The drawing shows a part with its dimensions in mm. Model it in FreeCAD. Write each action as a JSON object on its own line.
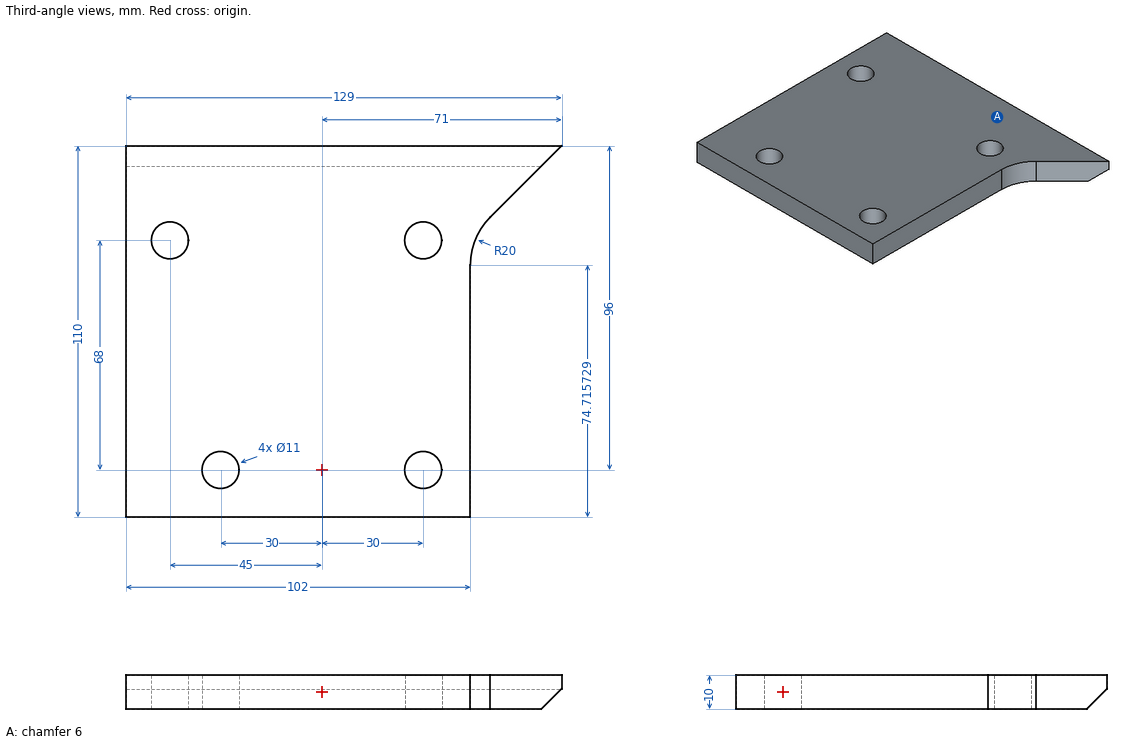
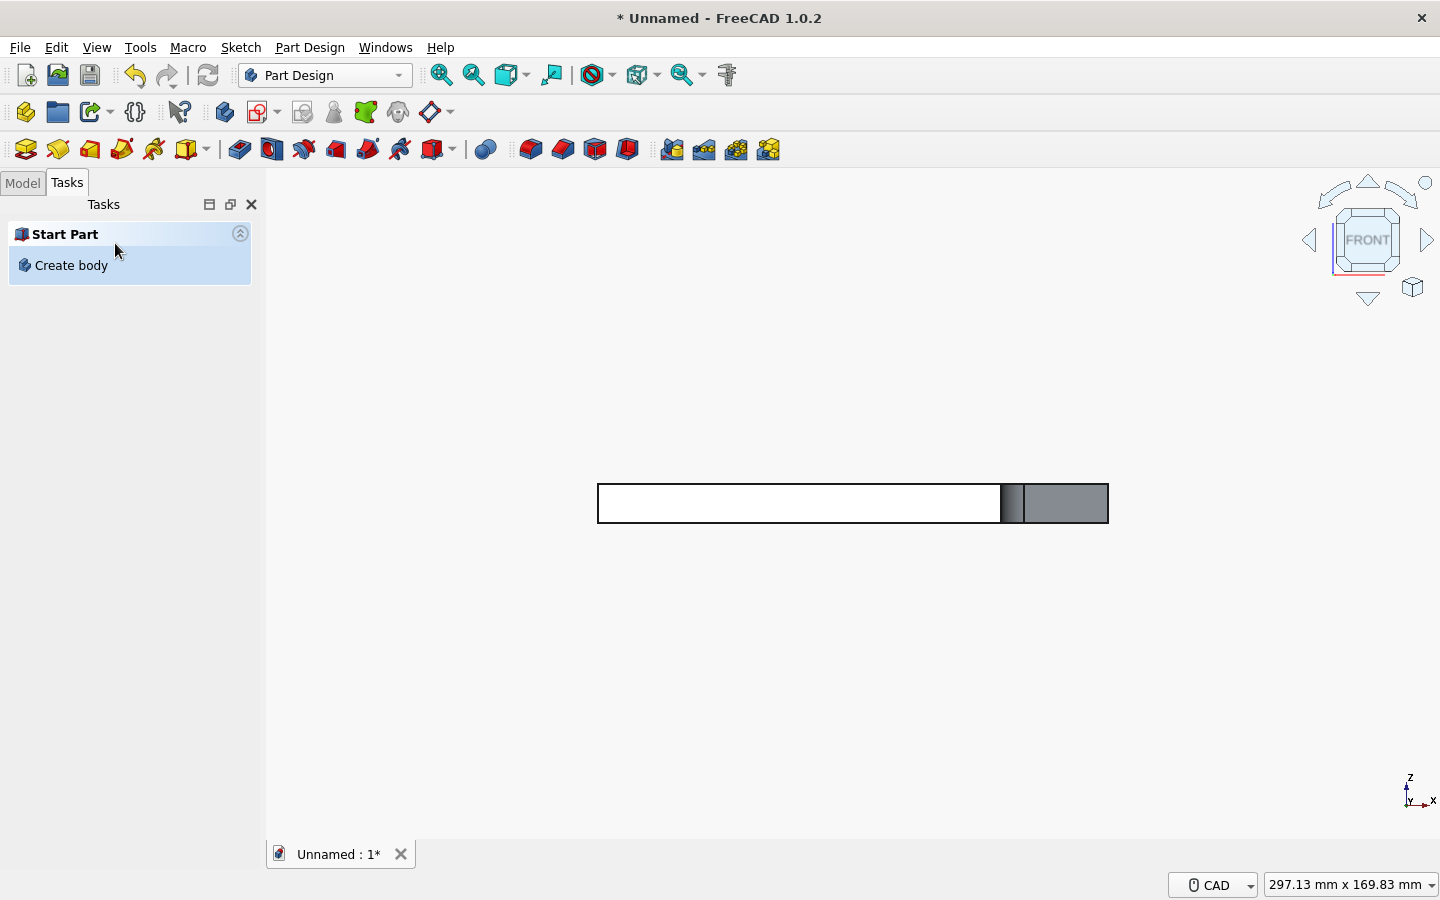
{"action": "key", "text": "3"}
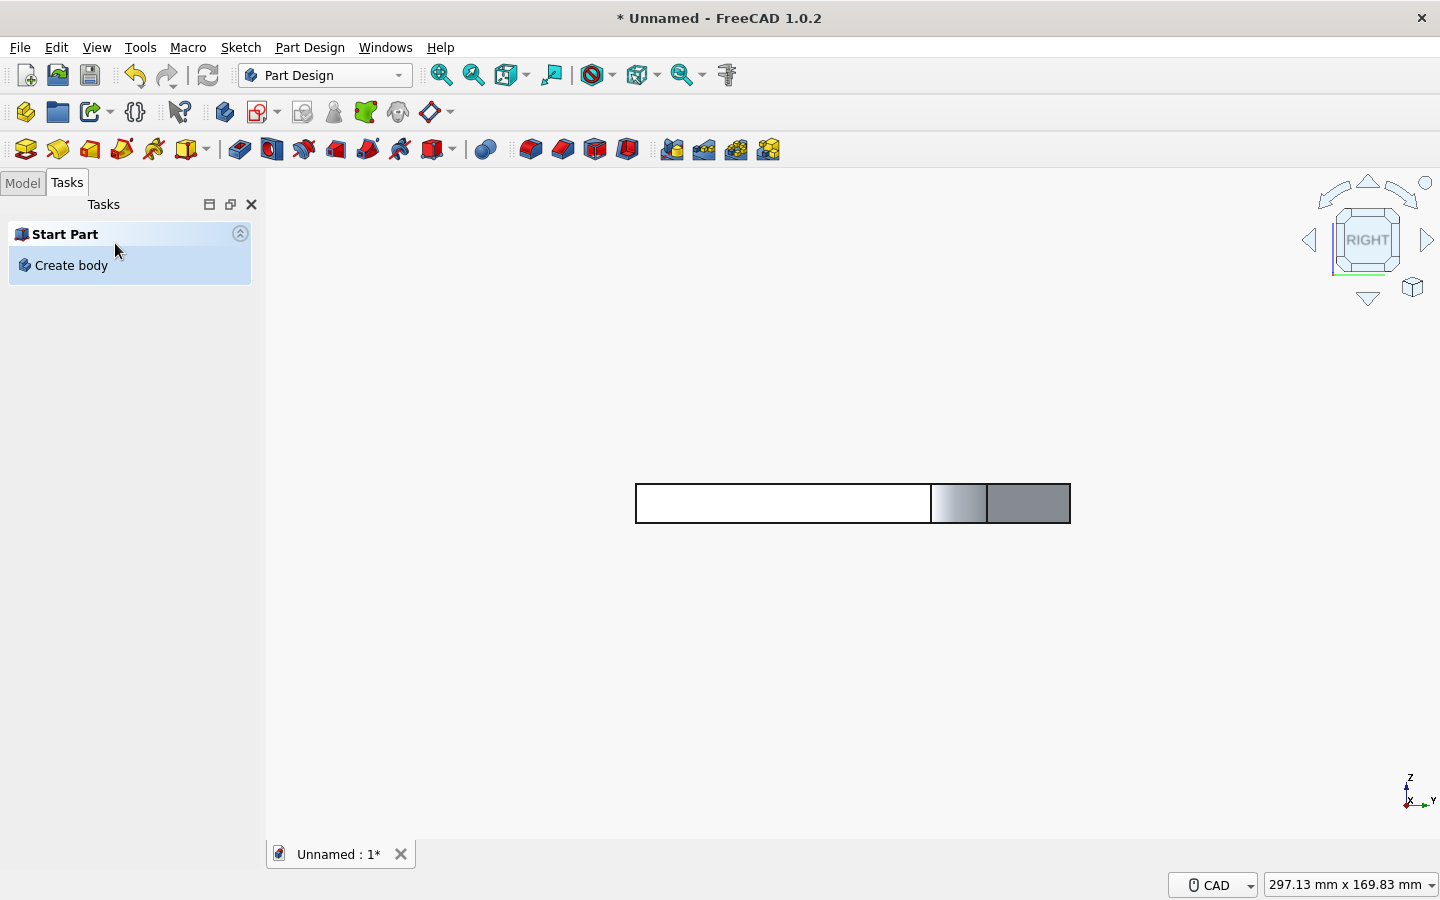
{"action": "key", "text": "v f"}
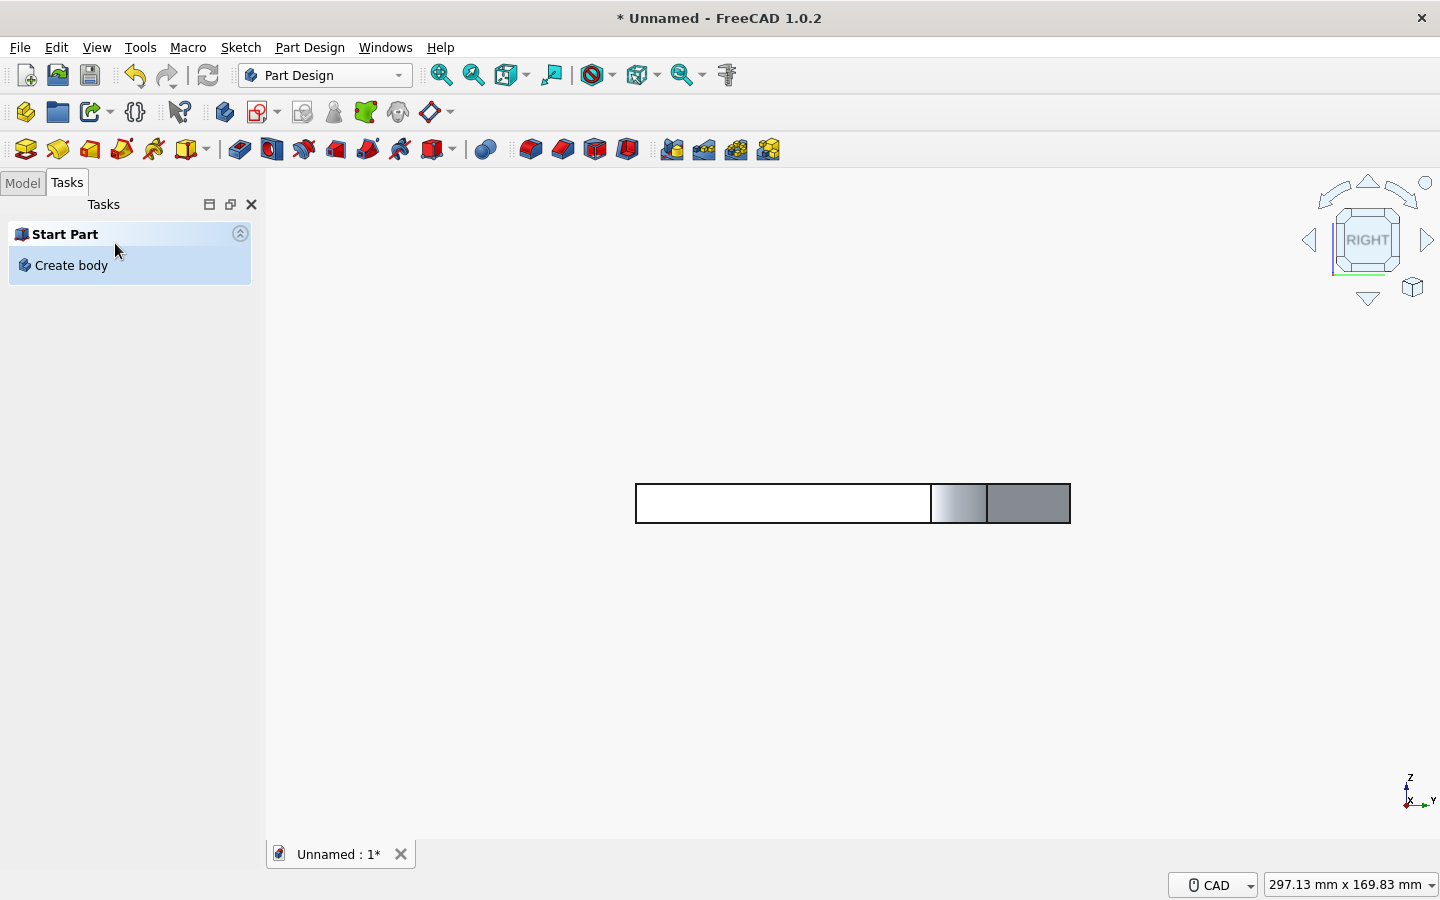
{"action": "key", "text": "5"}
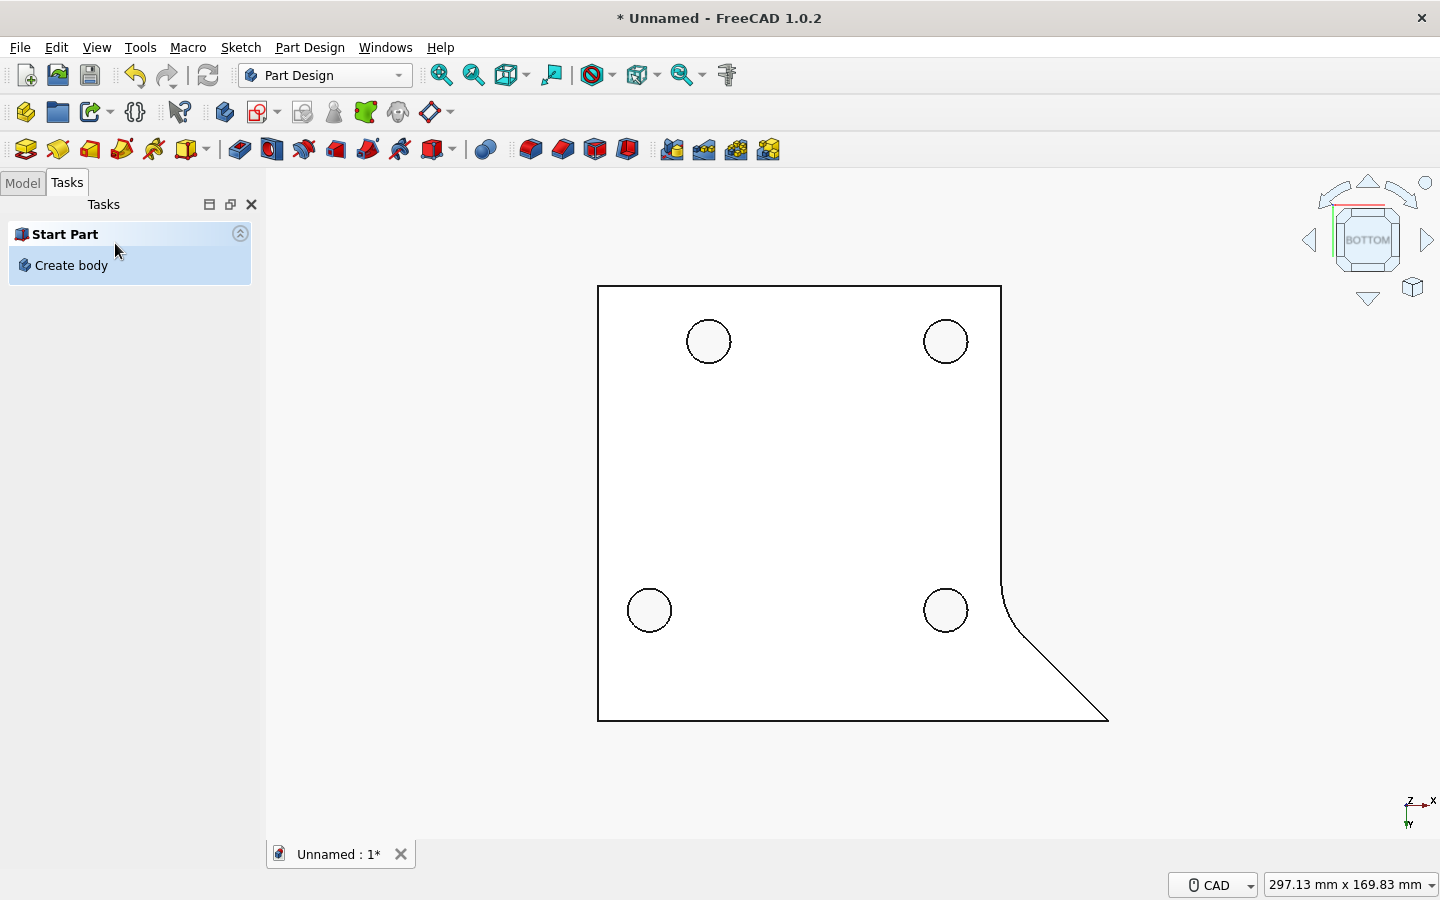
{"action": "left_click", "coordinate": [853, 720]}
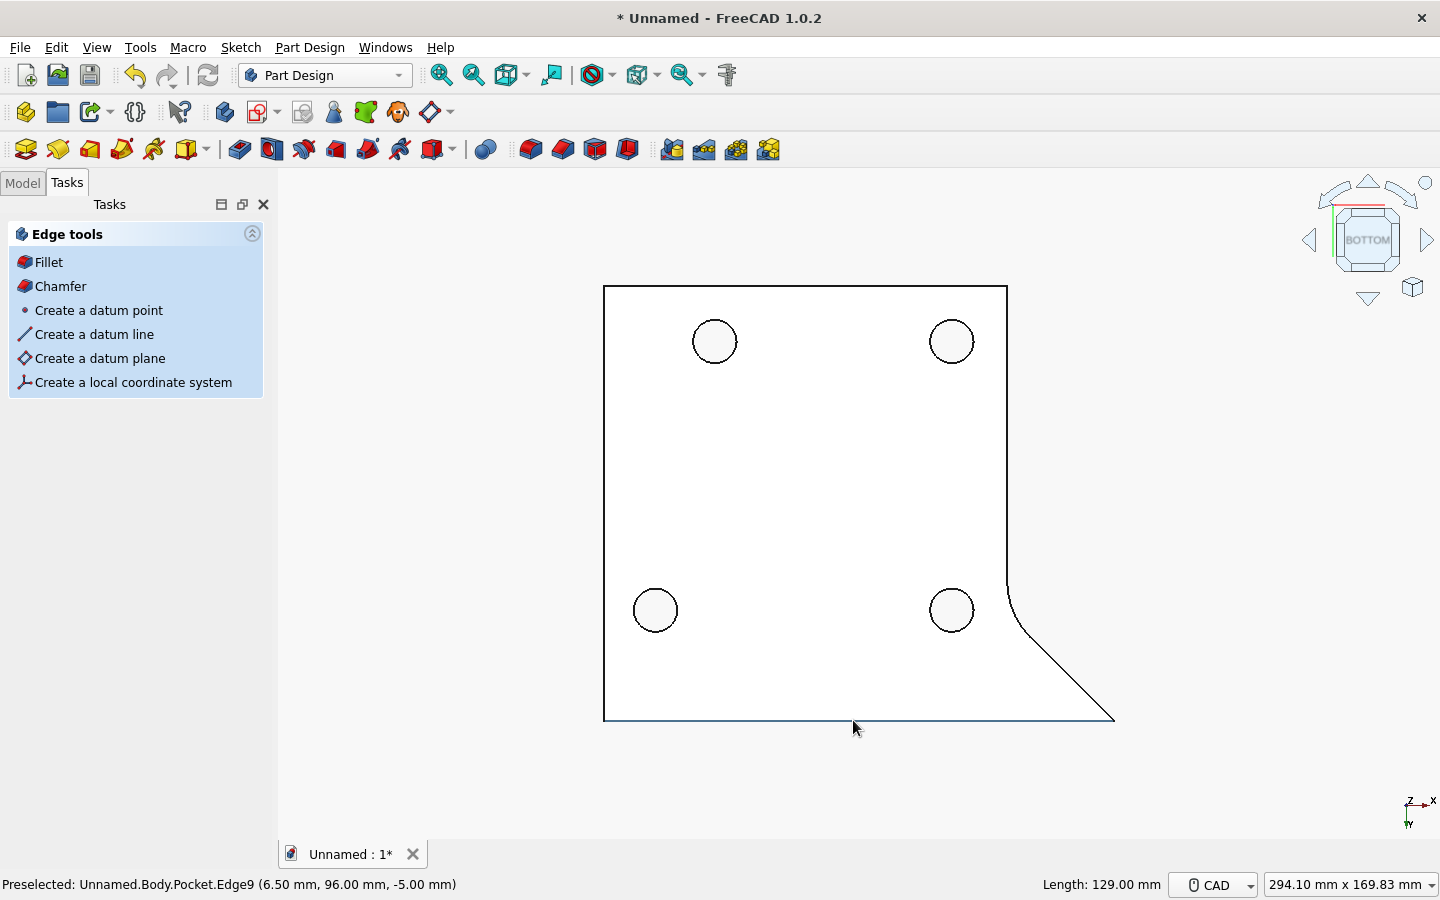
{"action": "left_click", "coordinate": [564, 150]}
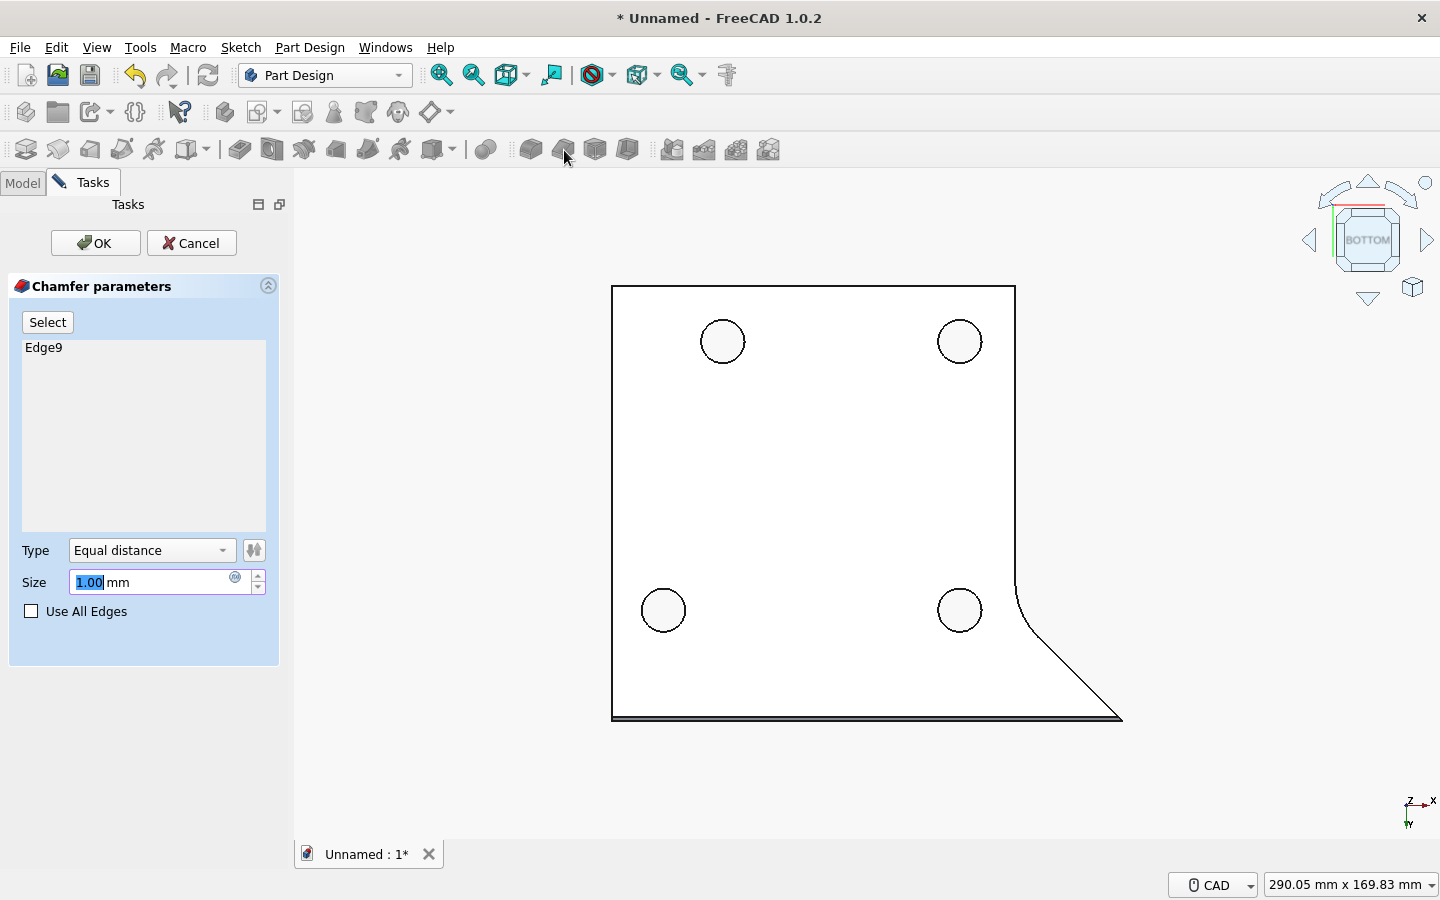
{"action": "type", "text": "6"}
{"action": "key", "text": "Tab"}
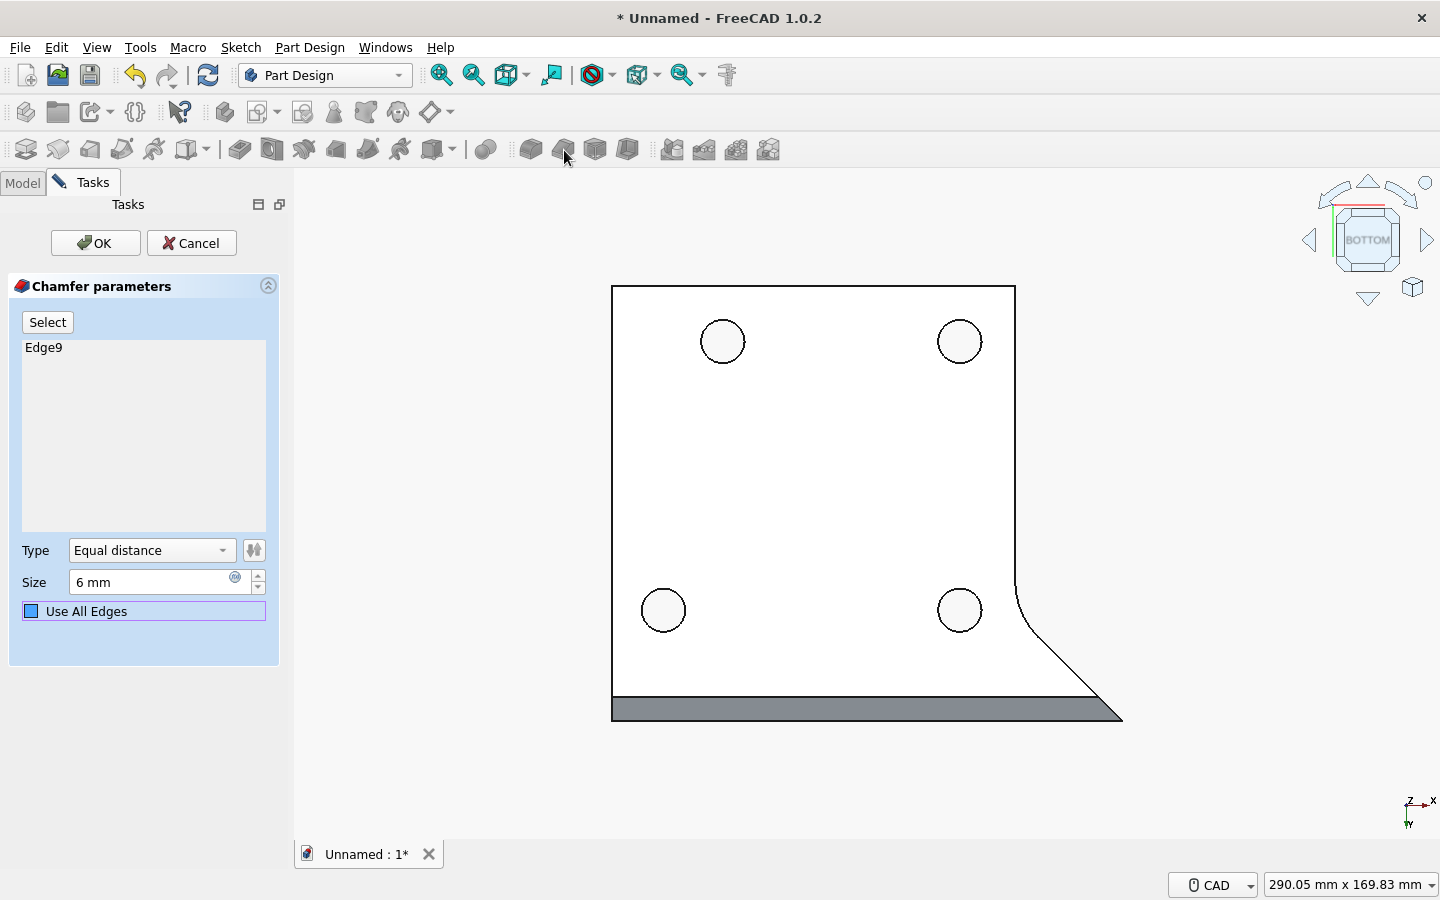
{"action": "left_click", "coordinate": [96, 243]}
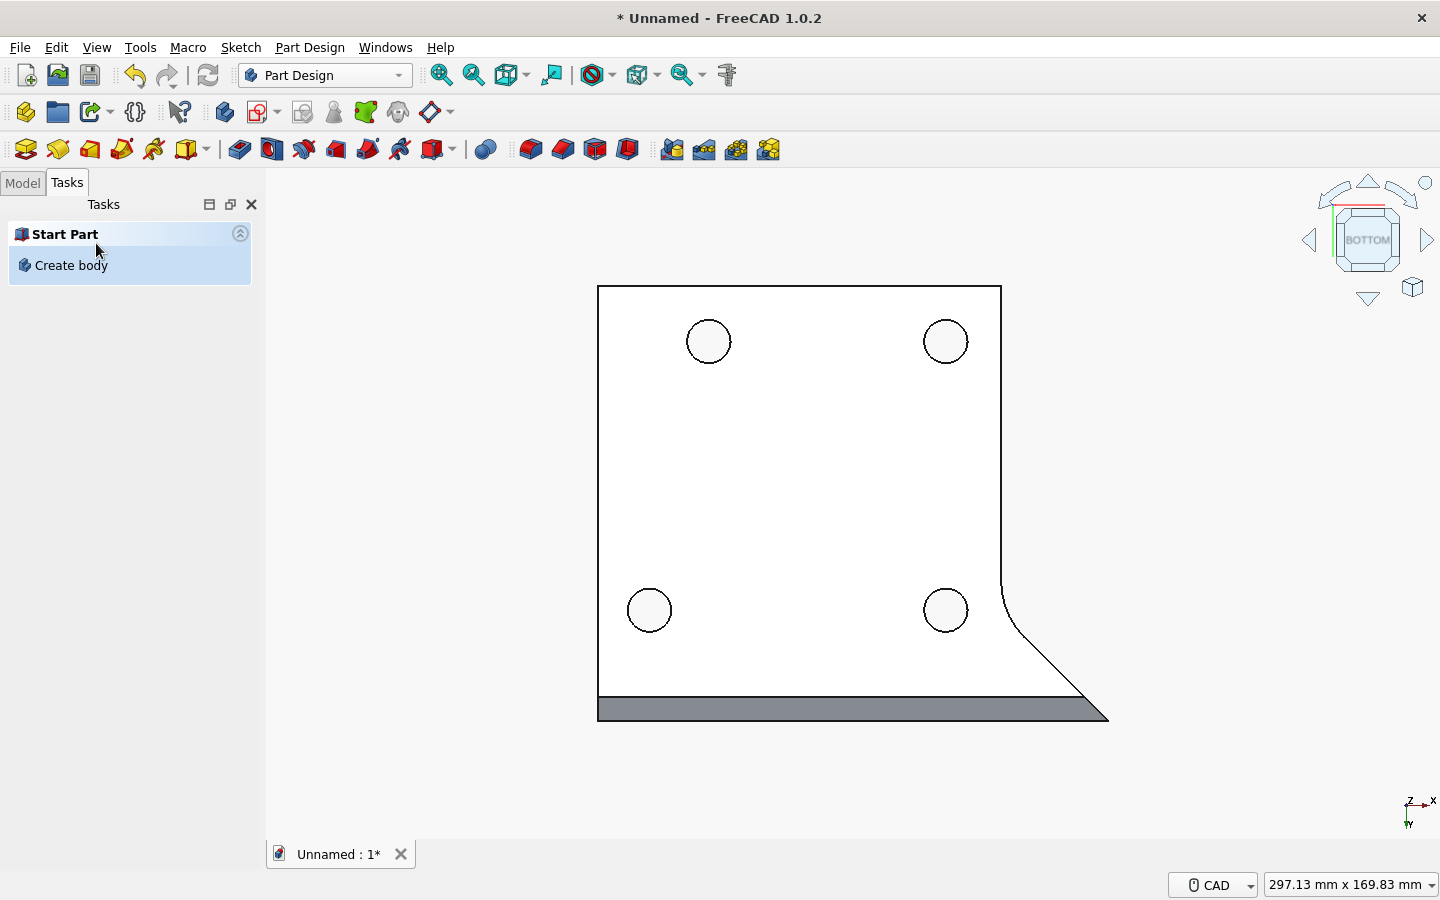
{"action": "key", "text": "0"}